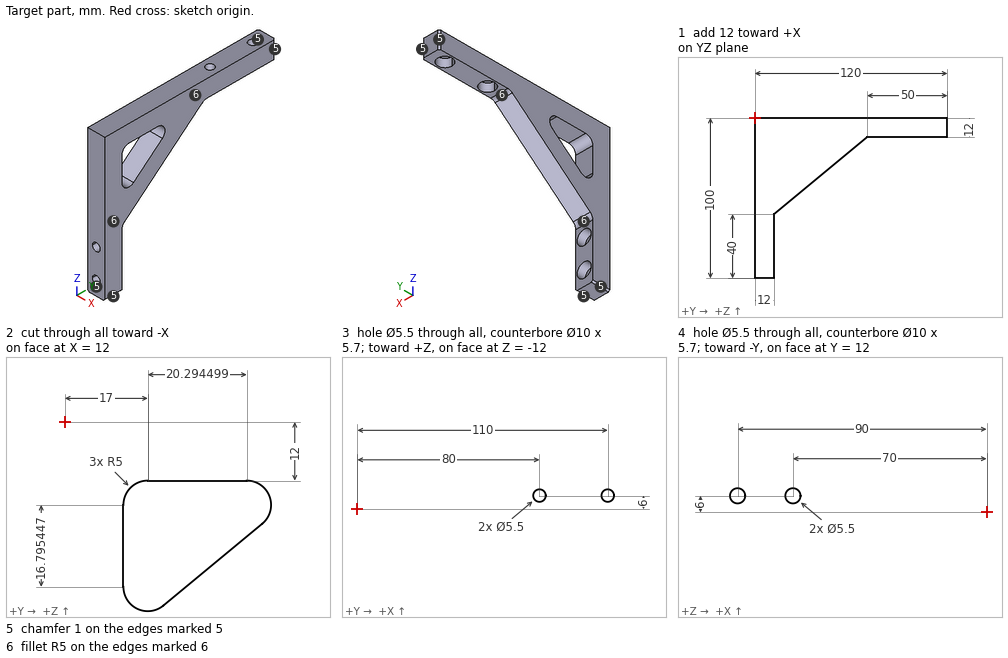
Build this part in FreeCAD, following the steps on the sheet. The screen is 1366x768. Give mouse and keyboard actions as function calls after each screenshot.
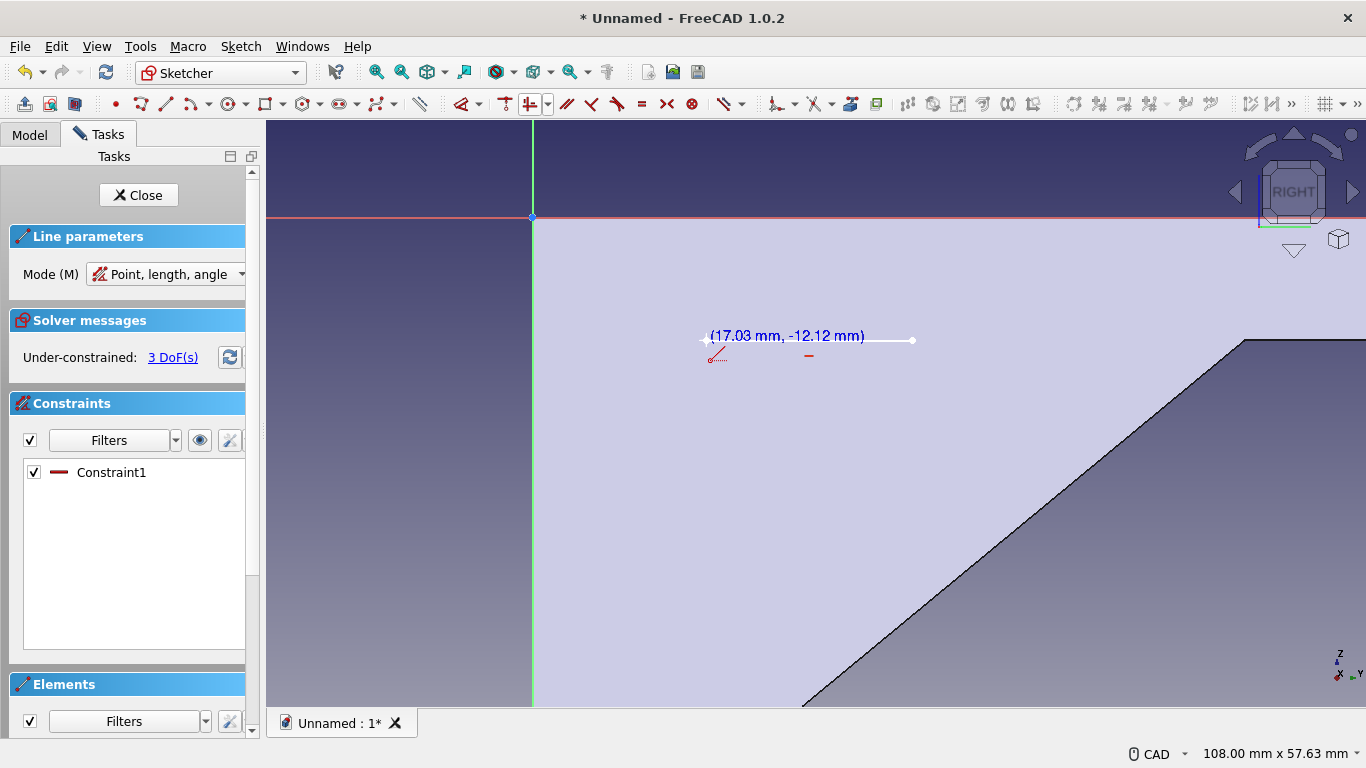
click(655, 391)
click(655, 562)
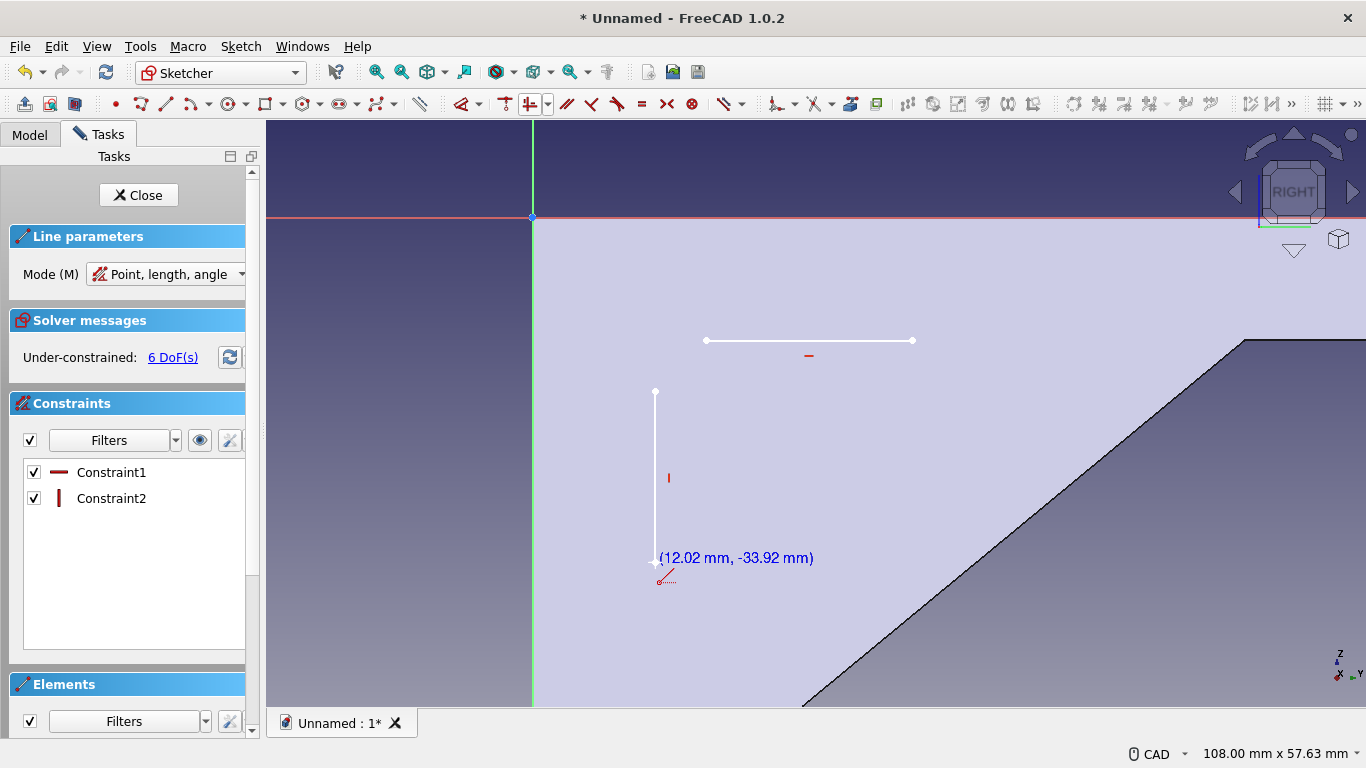
click(738, 601)
click(945, 430)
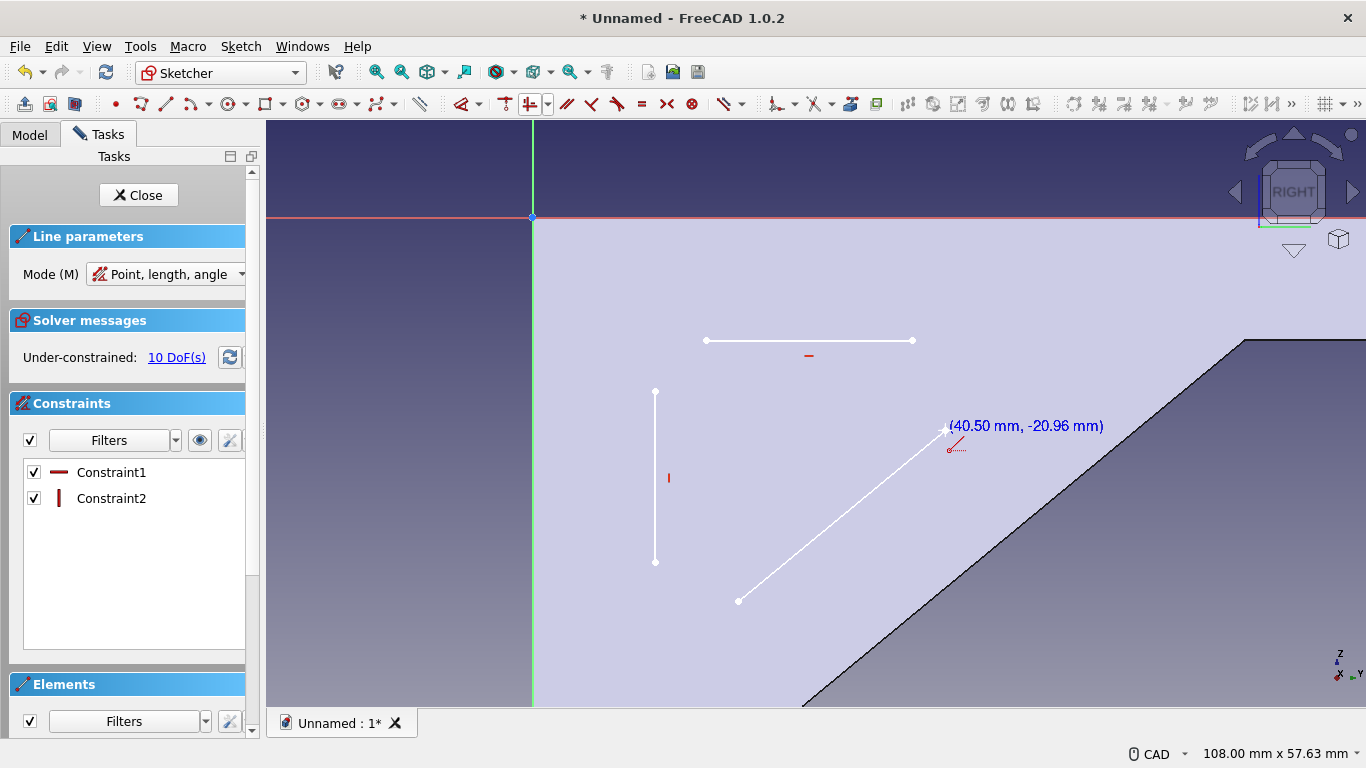
key(g)
key(3)
key(a)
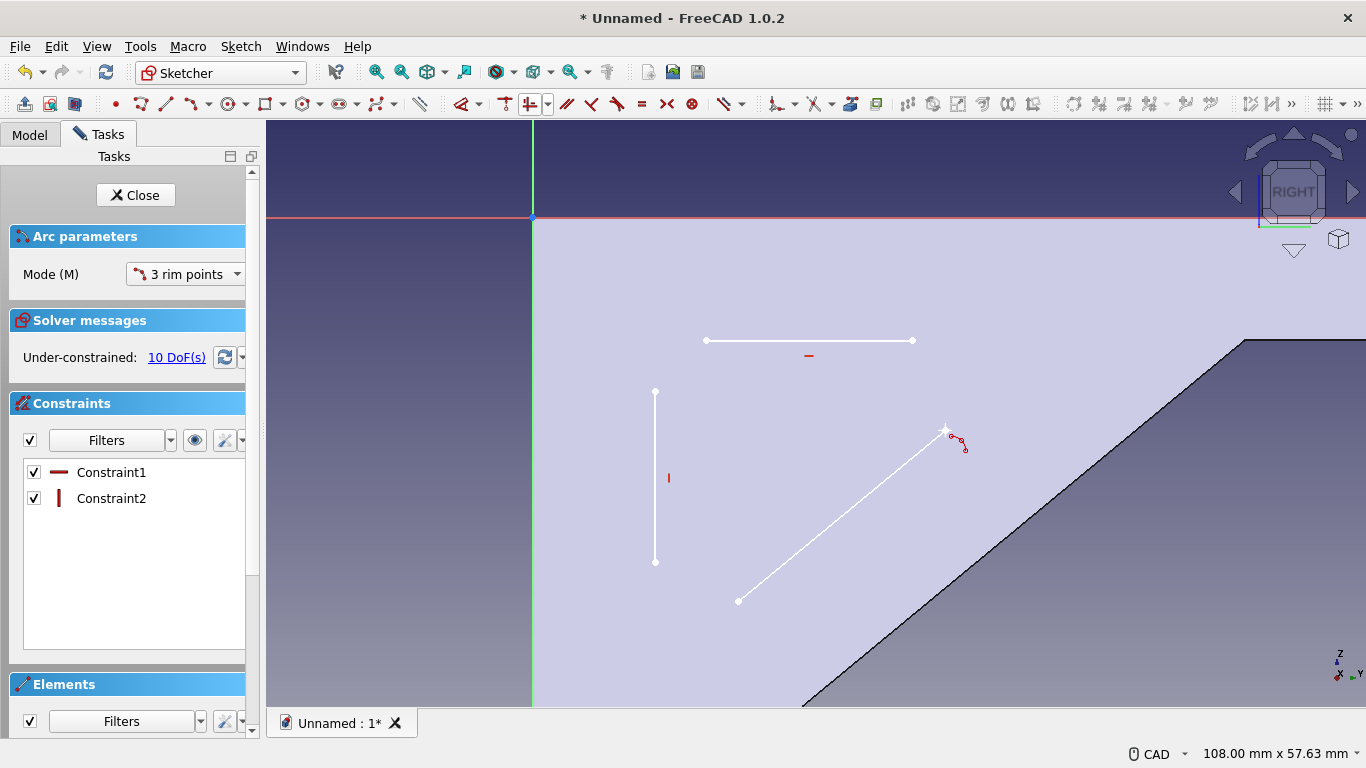
click(706, 341)
click(655, 392)
click(670, 355)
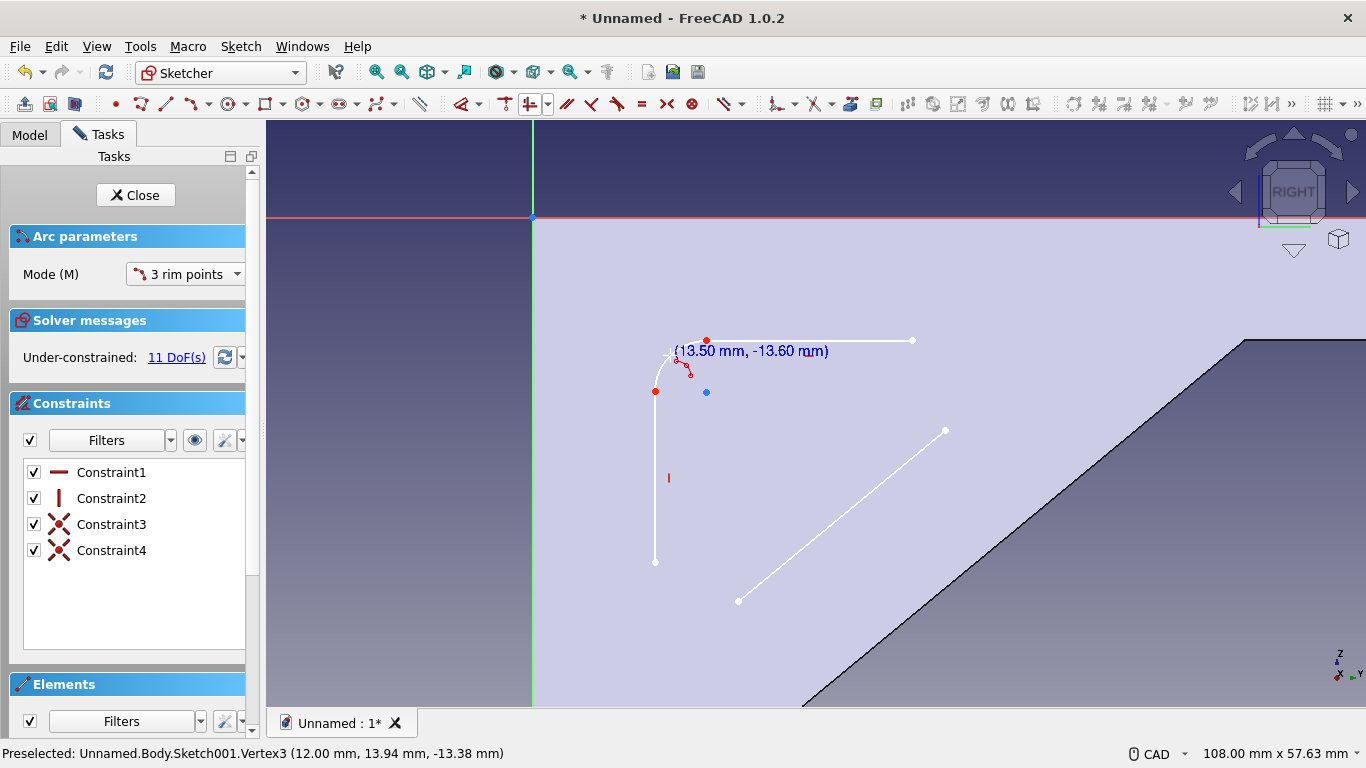
click(655, 563)
click(738, 602)
click(684, 608)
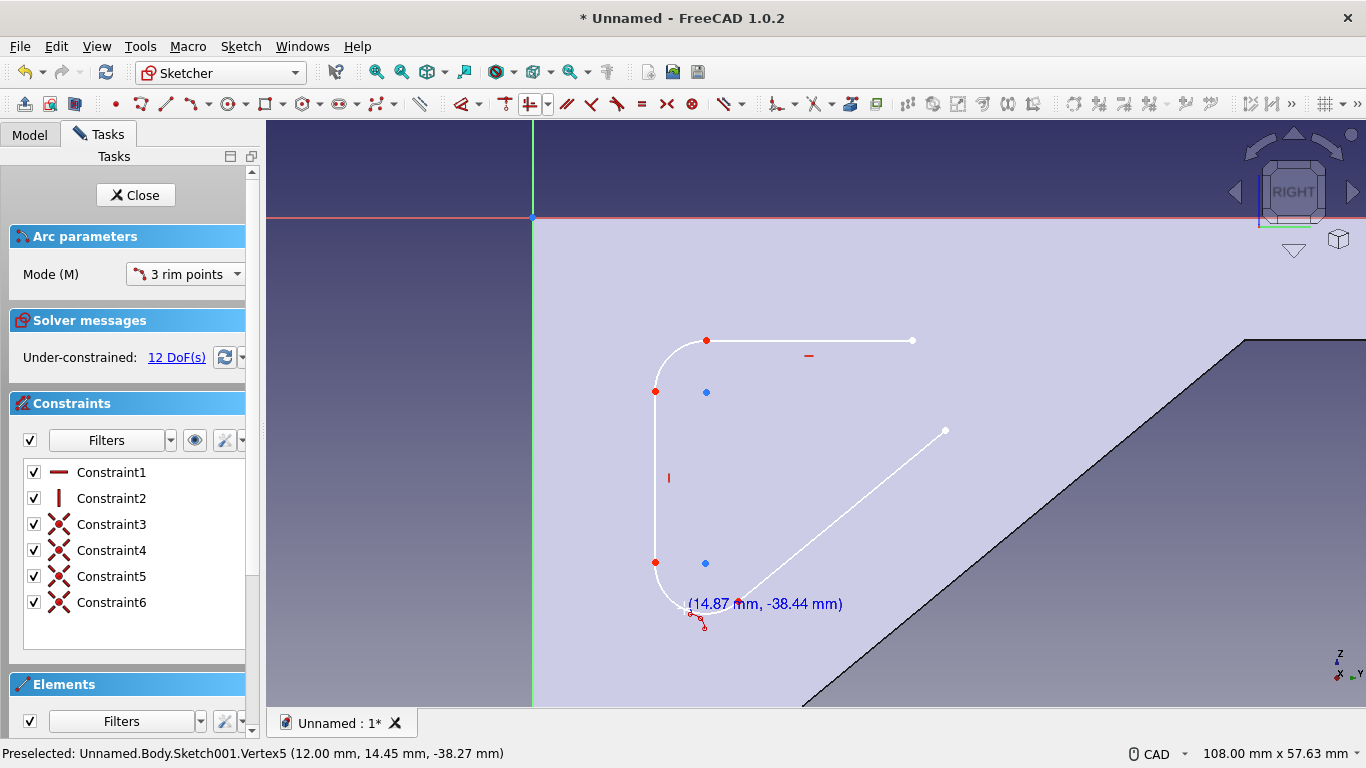
click(945, 431)
click(912, 341)
click(960, 373)
key(Escape)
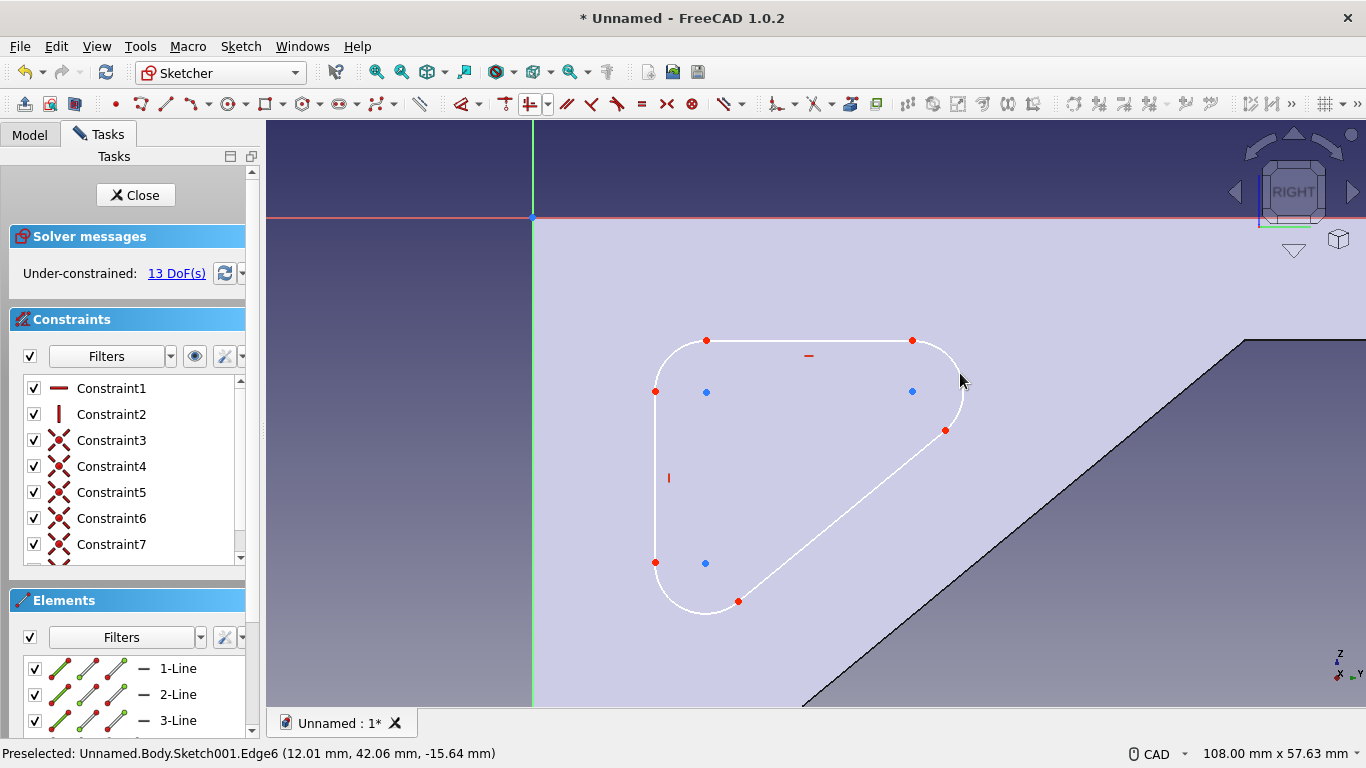
click(850, 341)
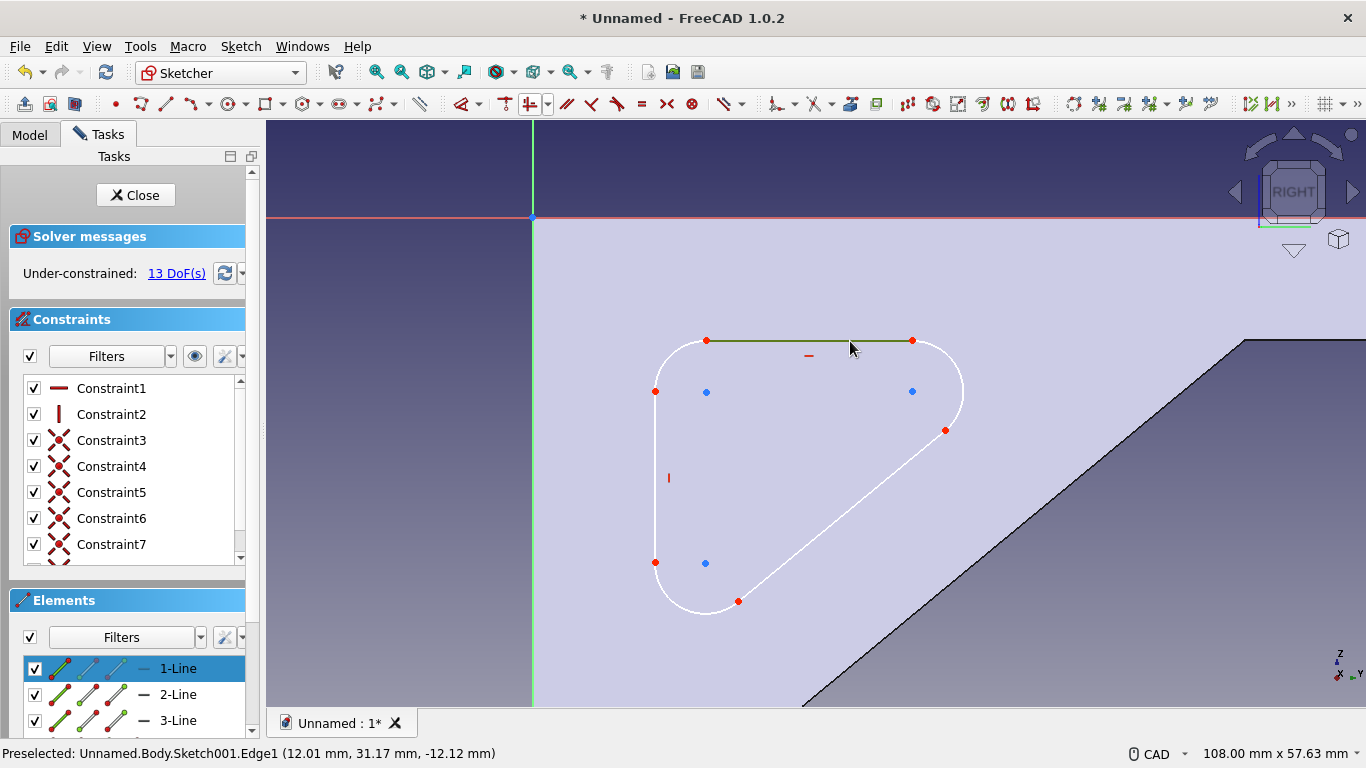
click(683, 347)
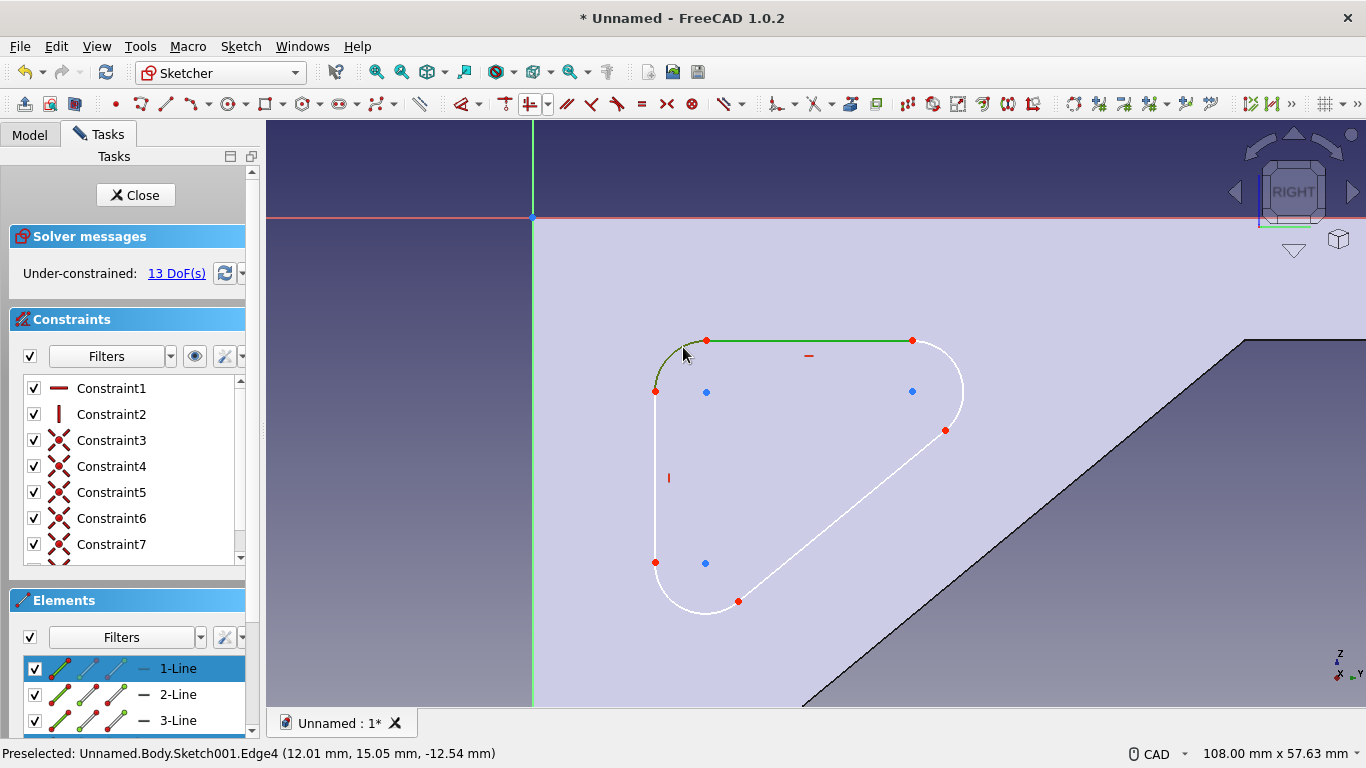
click(617, 104)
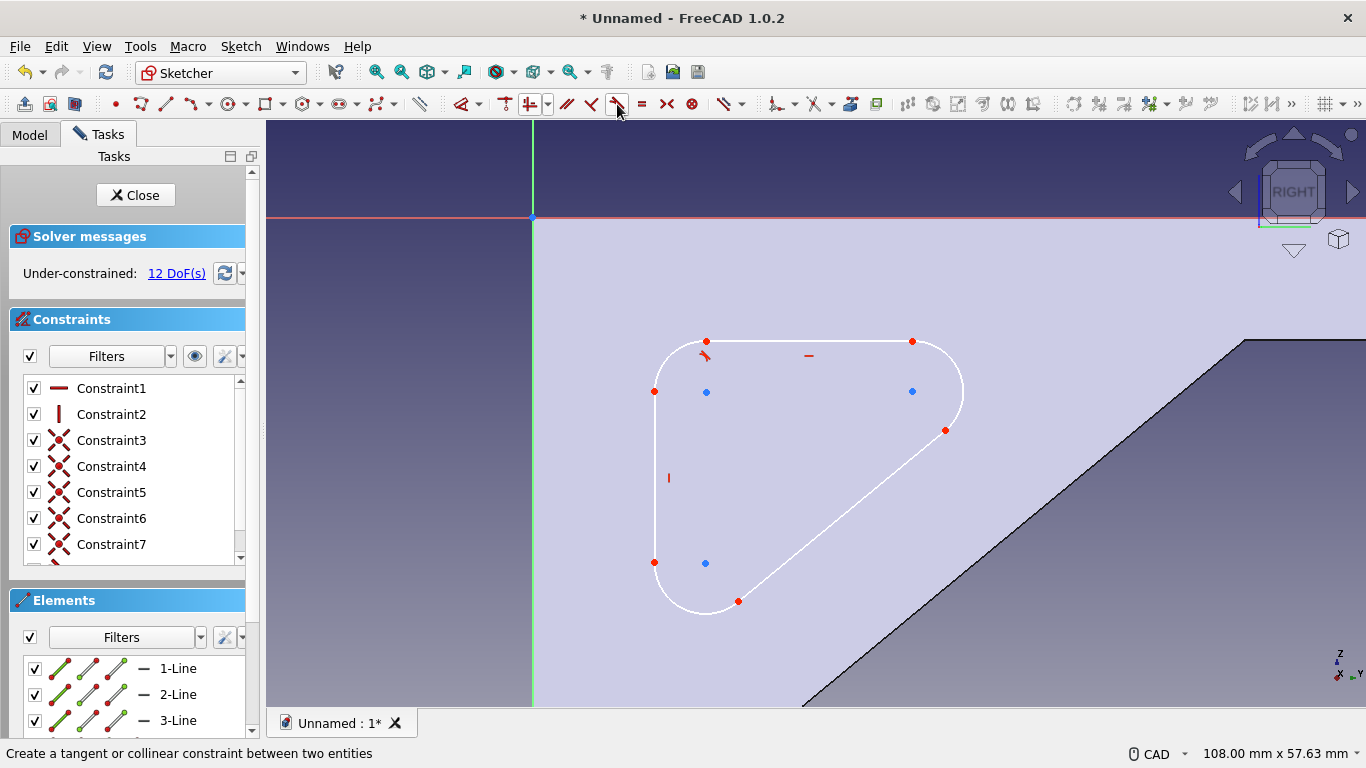
click(850, 341)